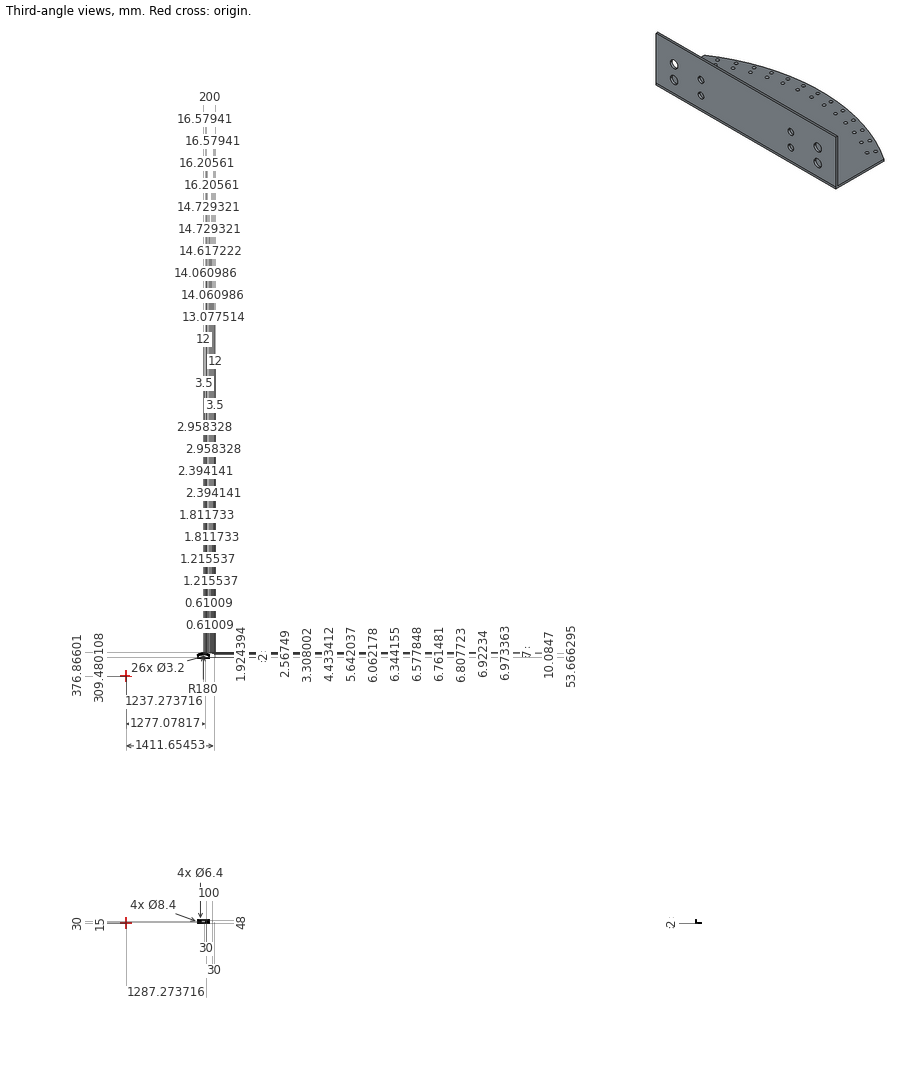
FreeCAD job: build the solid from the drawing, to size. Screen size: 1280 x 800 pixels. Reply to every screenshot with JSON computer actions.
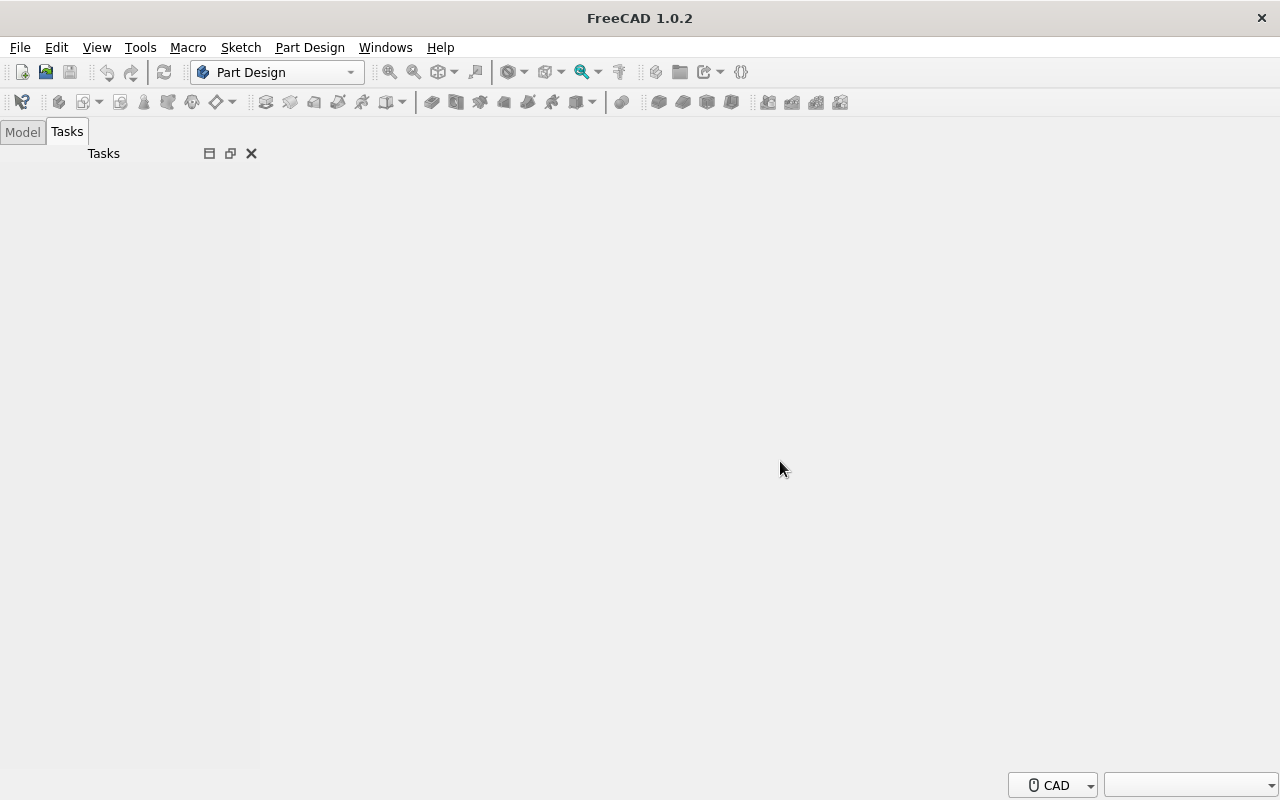
{"action": "key", "text": "ctrl+n"}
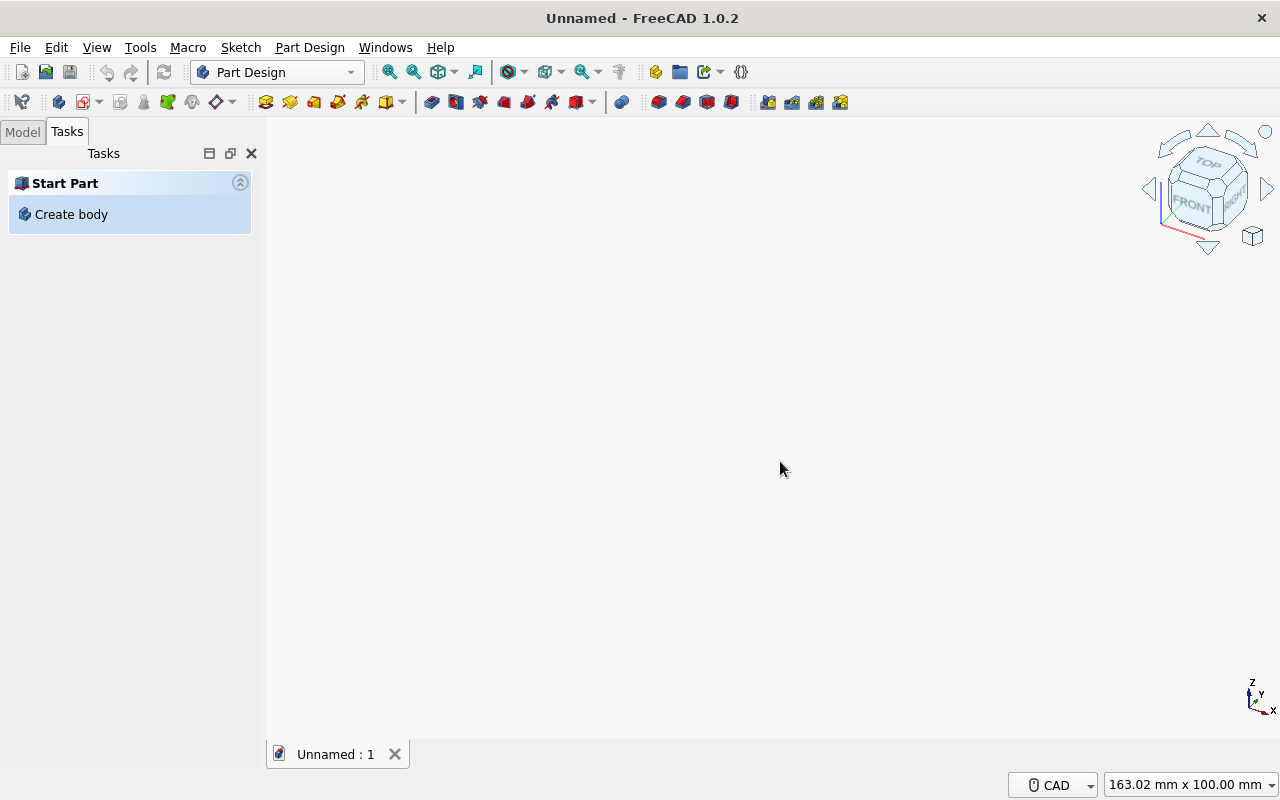
{"action": "left_click", "coordinate": [84, 102]}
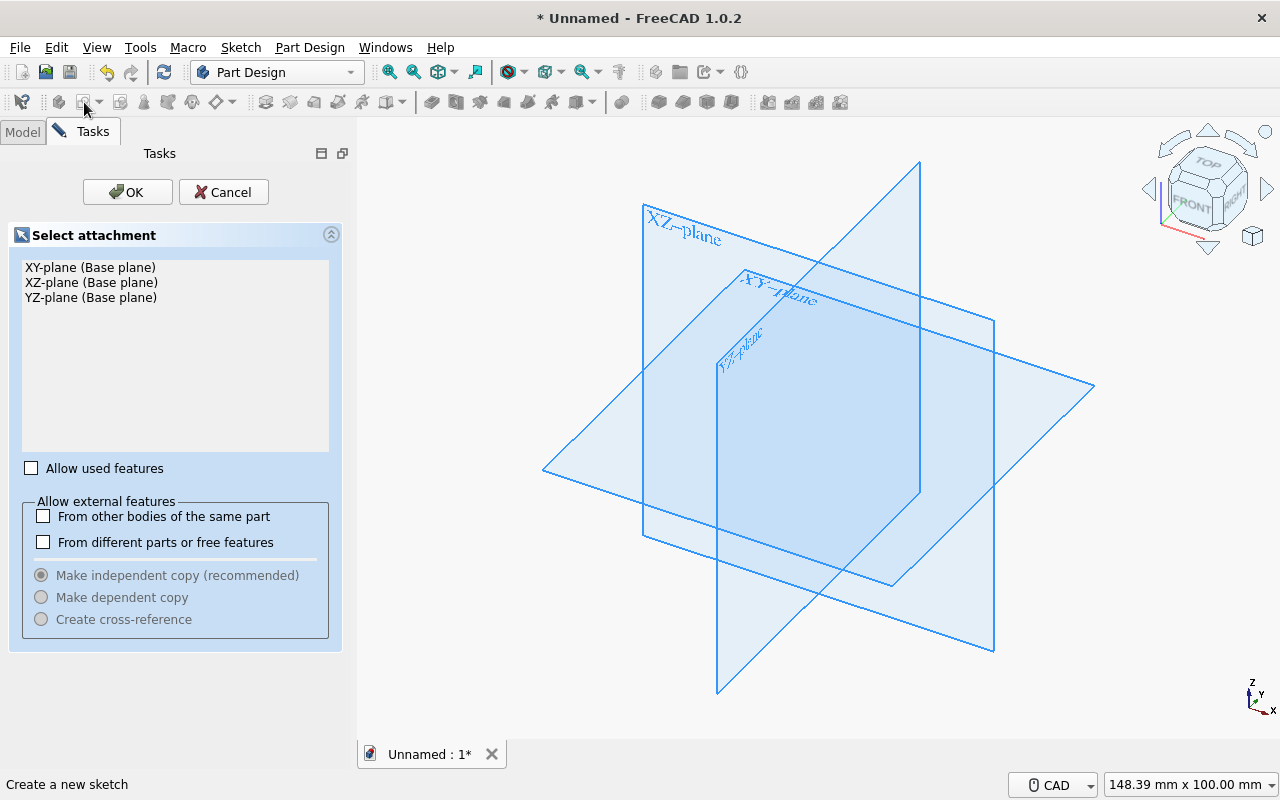
{"action": "left_click", "coordinate": [82, 268]}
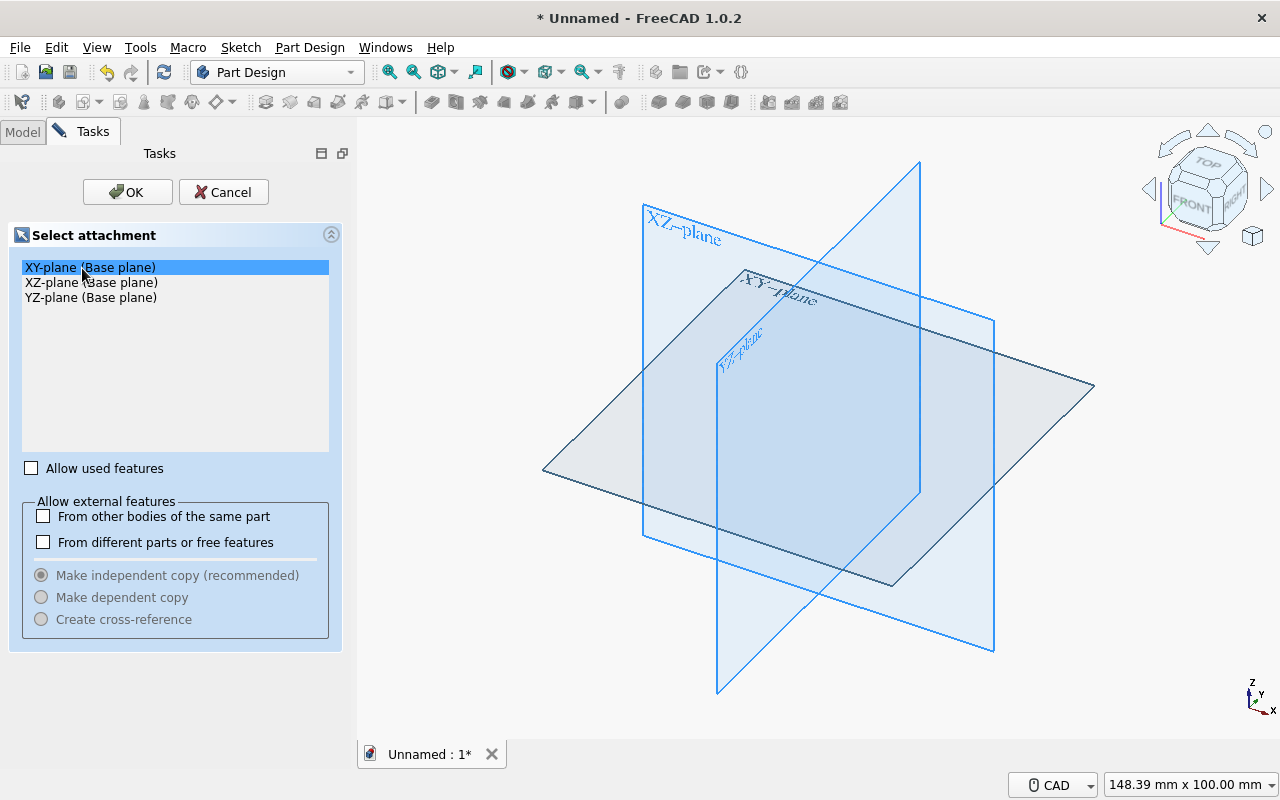
{"action": "left_click", "coordinate": [128, 192]}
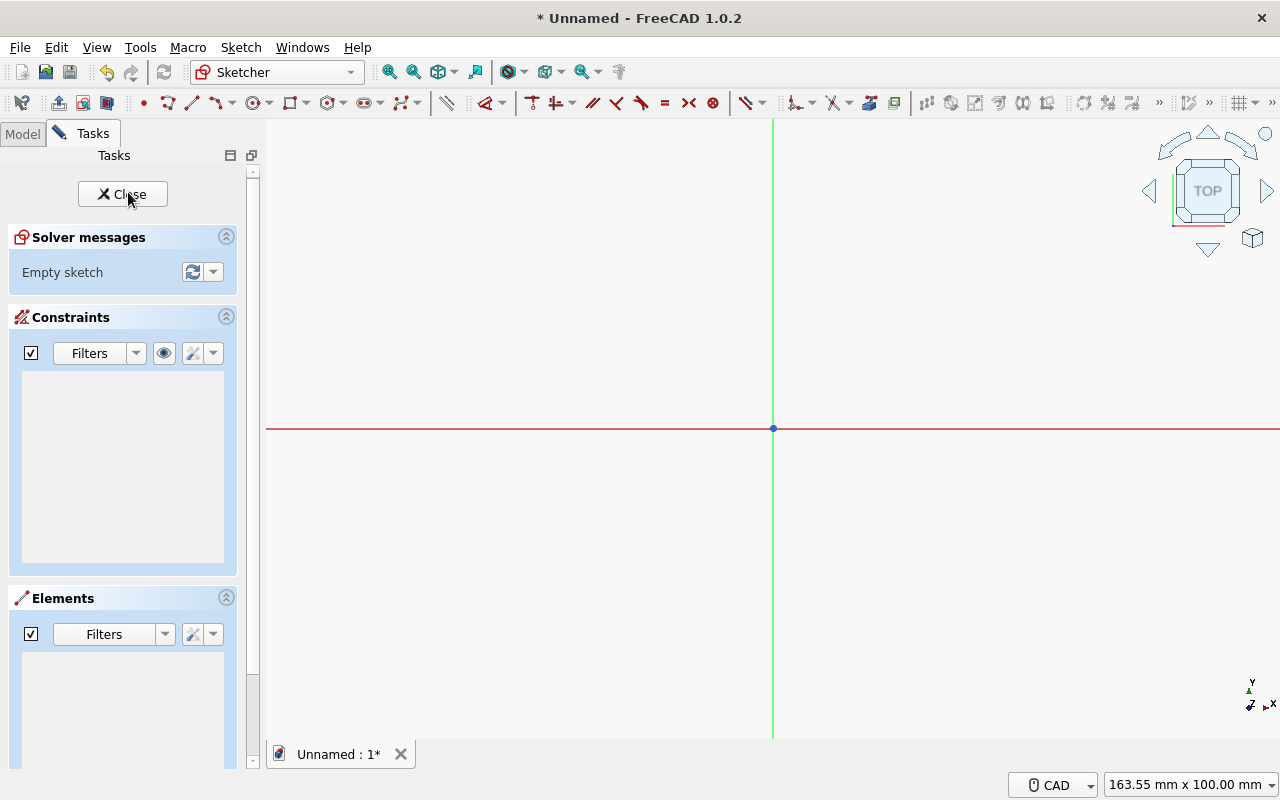
{"action": "scroll", "coordinate": [704, 429], "scroll_direction": "down", "scroll_amount": 5}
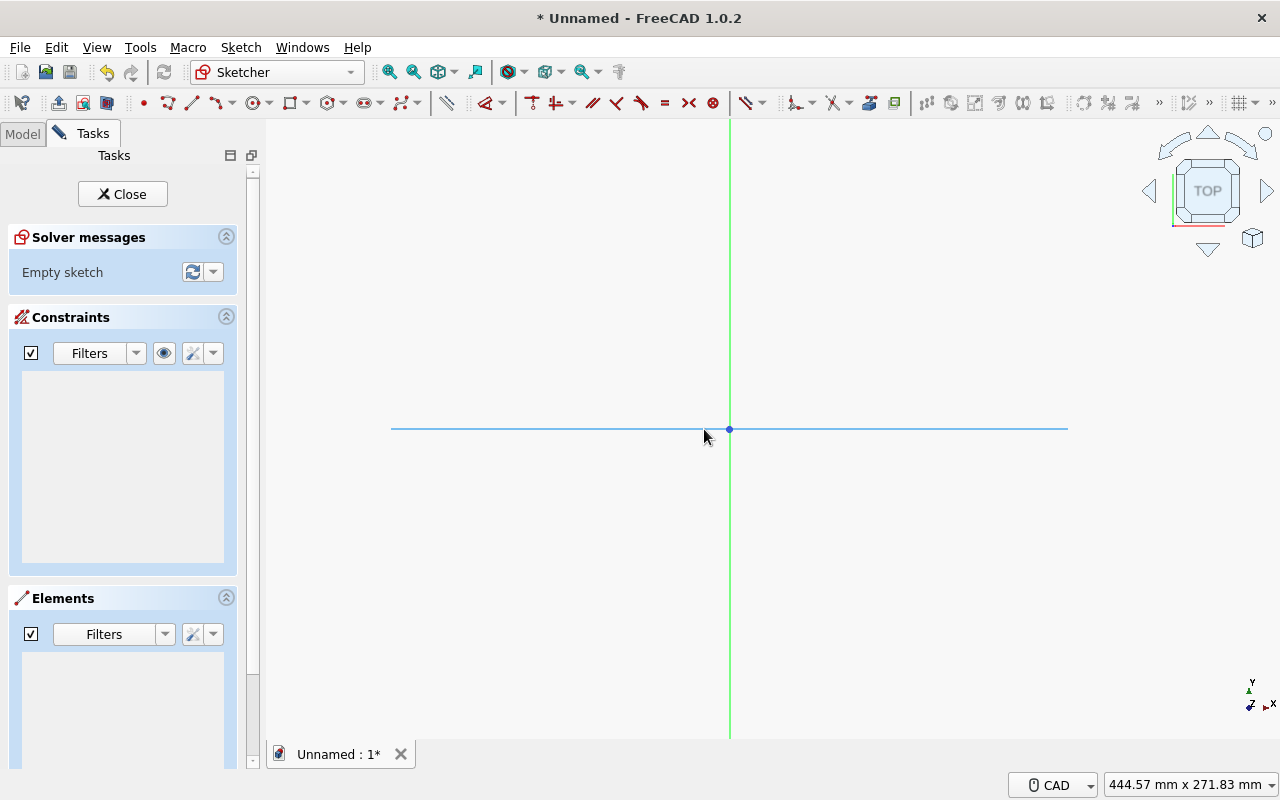
{"action": "scroll", "coordinate": [704, 429], "scroll_direction": "down", "scroll_amount": 5}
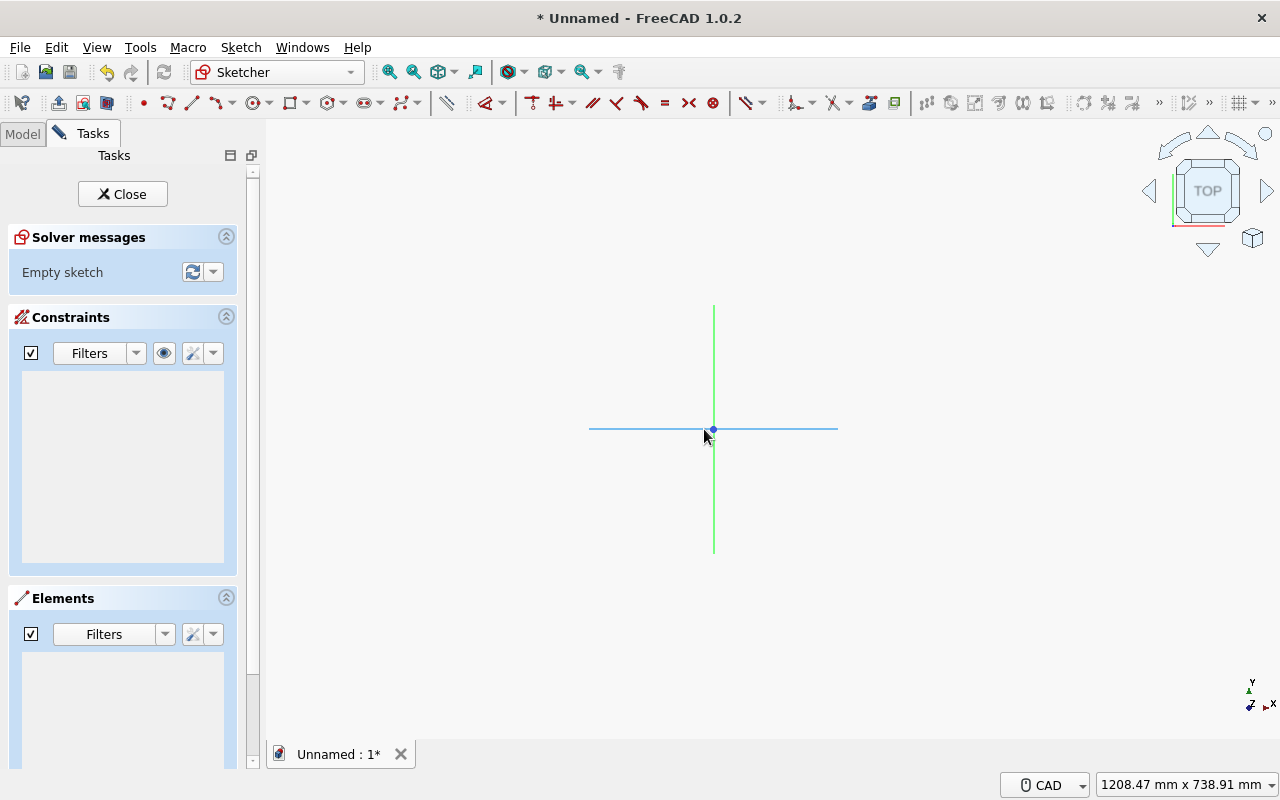
{"action": "scroll", "coordinate": [704, 429], "scroll_direction": "down", "scroll_amount": 5}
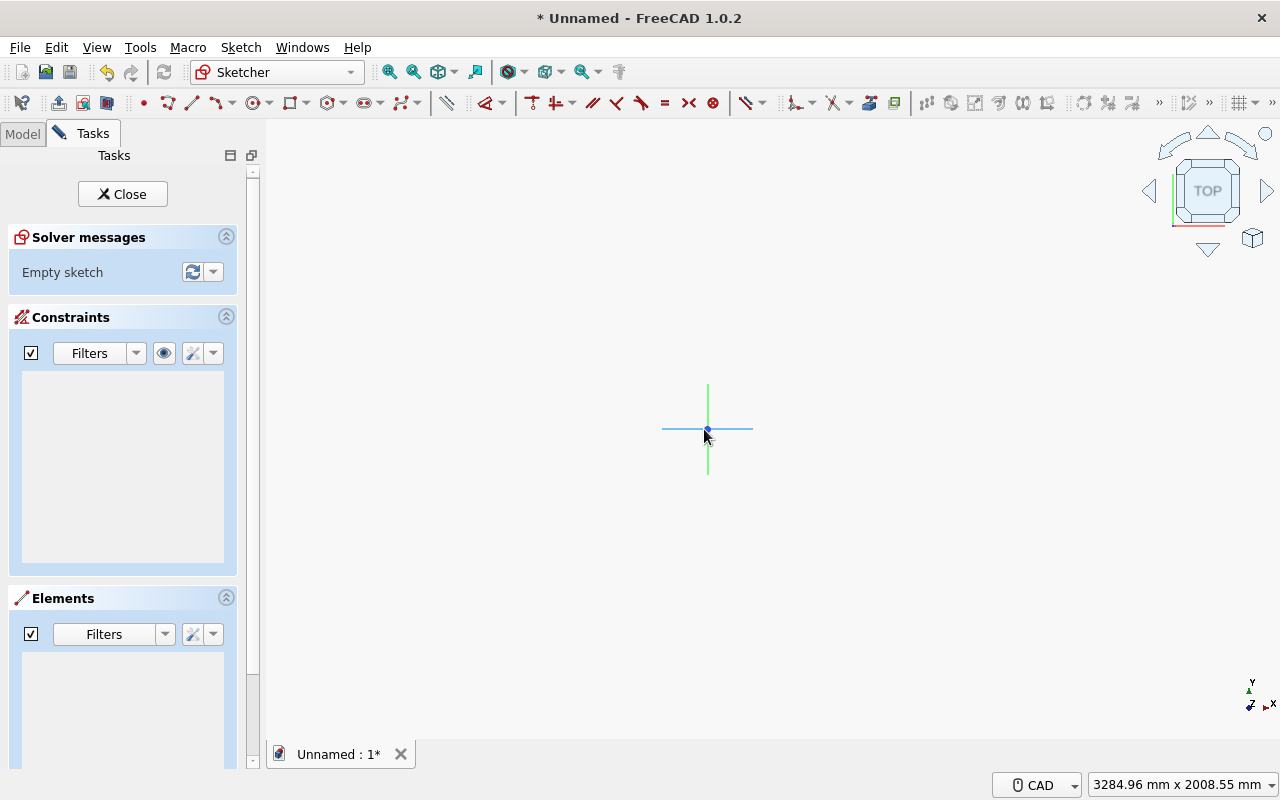
{"action": "scroll", "coordinate": [704, 429], "scroll_direction": "down", "scroll_amount": 5}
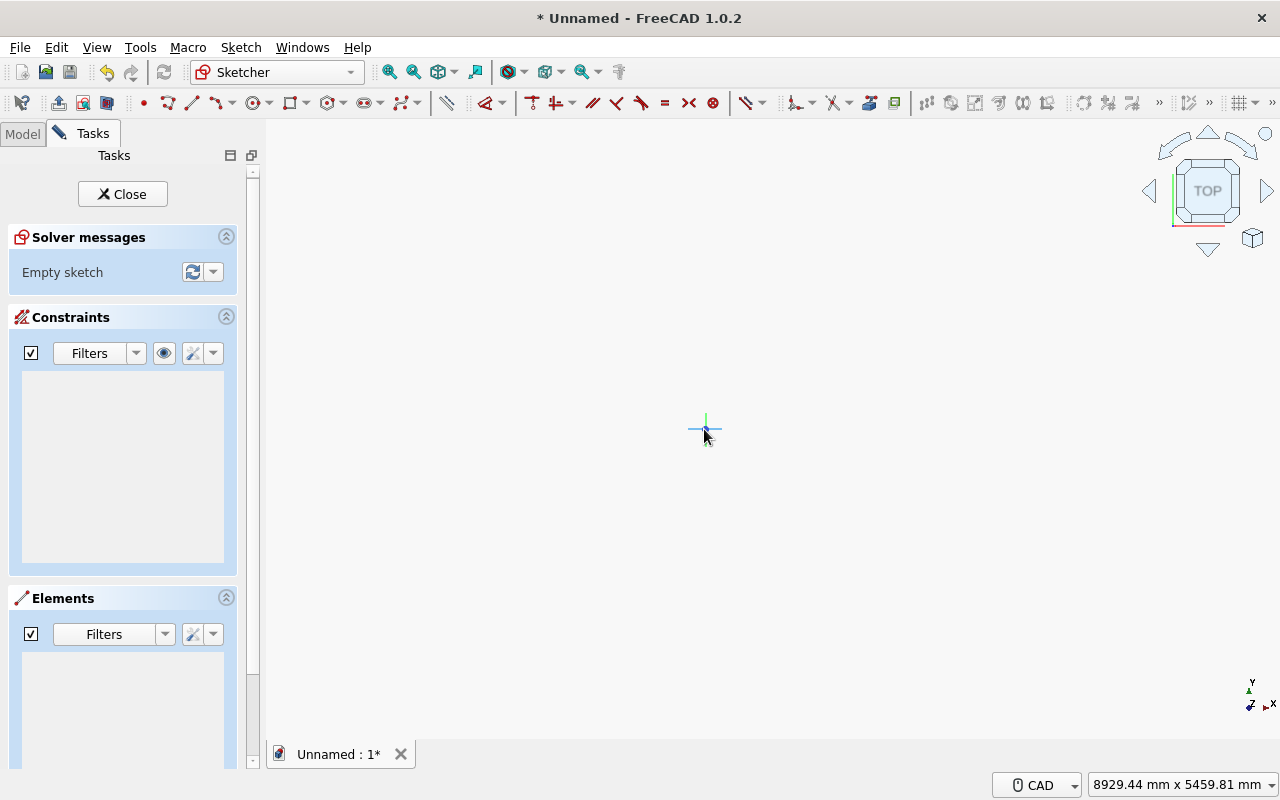
{"action": "scroll", "coordinate": [866, 388], "scroll_direction": "up", "scroll_amount": 15}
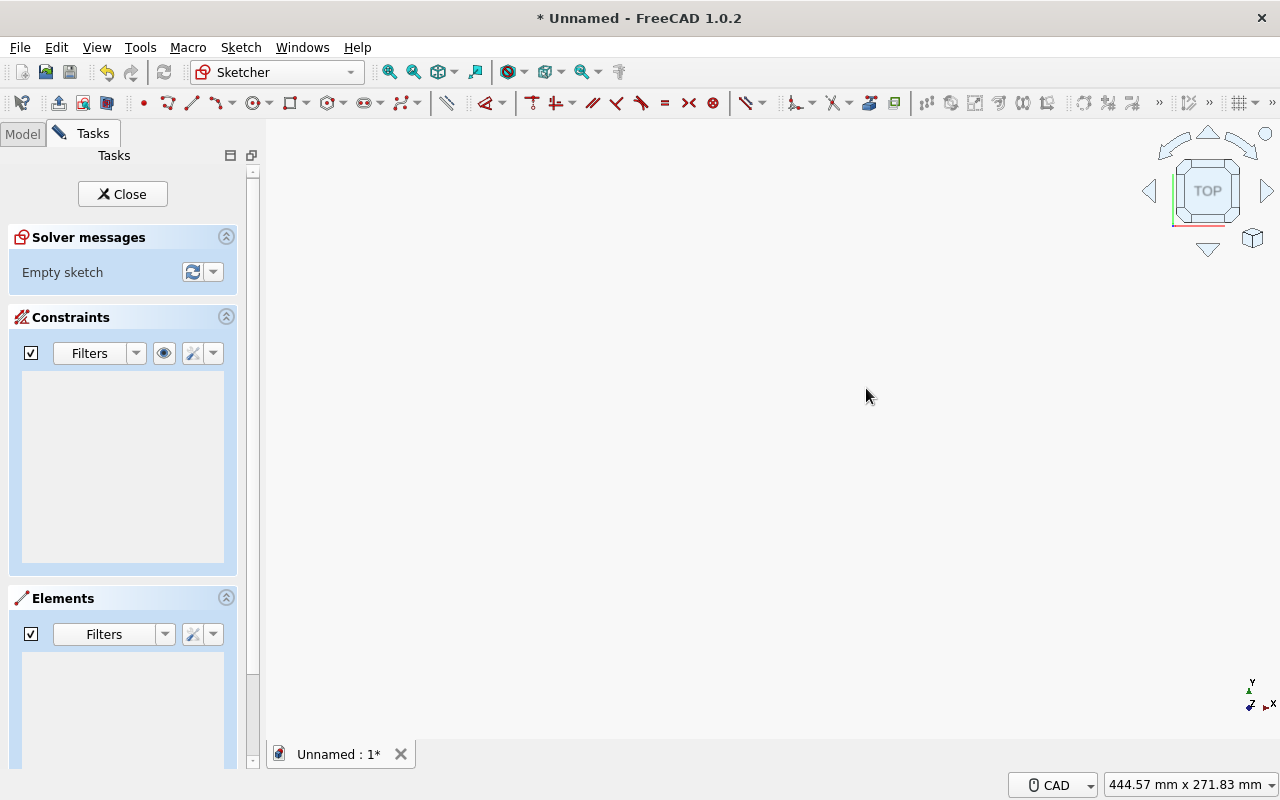
{"action": "key", "text": "g m"}